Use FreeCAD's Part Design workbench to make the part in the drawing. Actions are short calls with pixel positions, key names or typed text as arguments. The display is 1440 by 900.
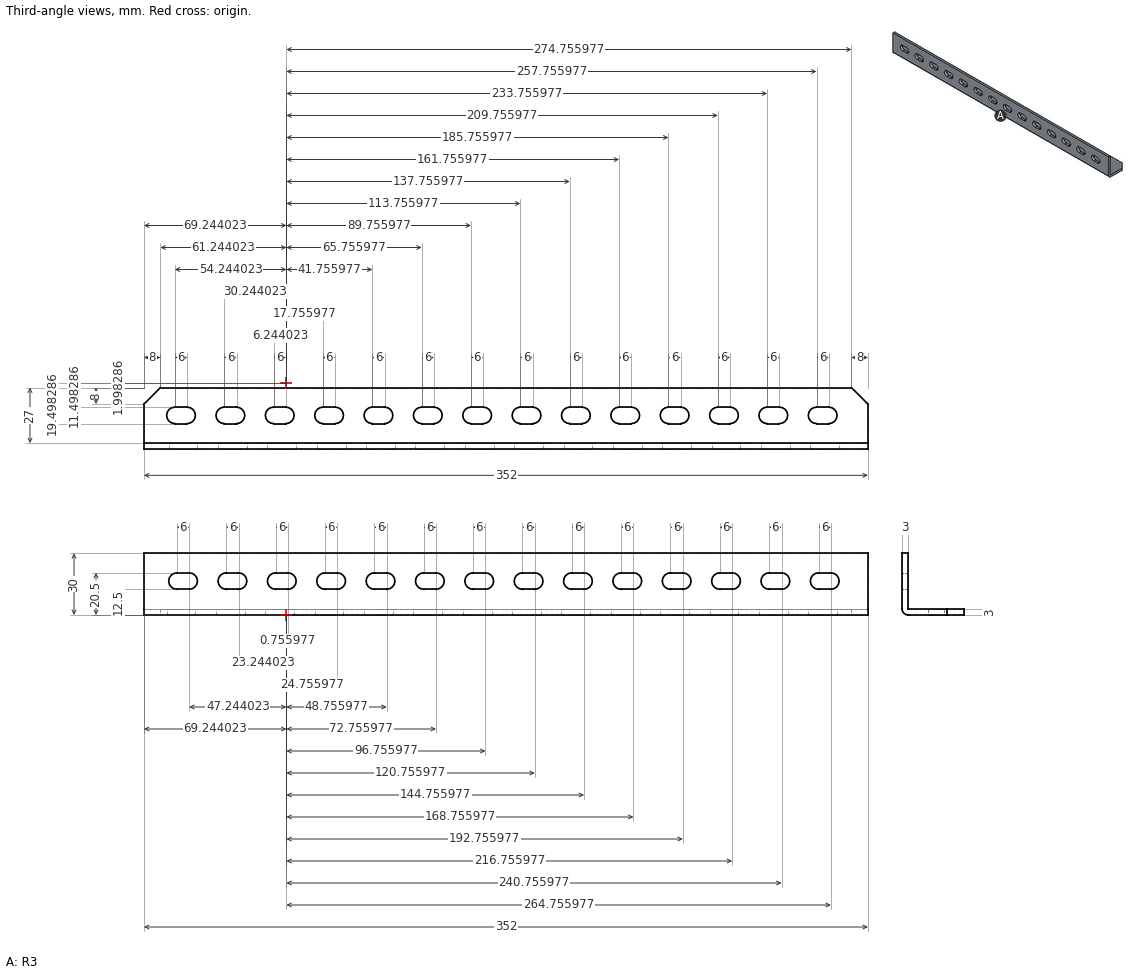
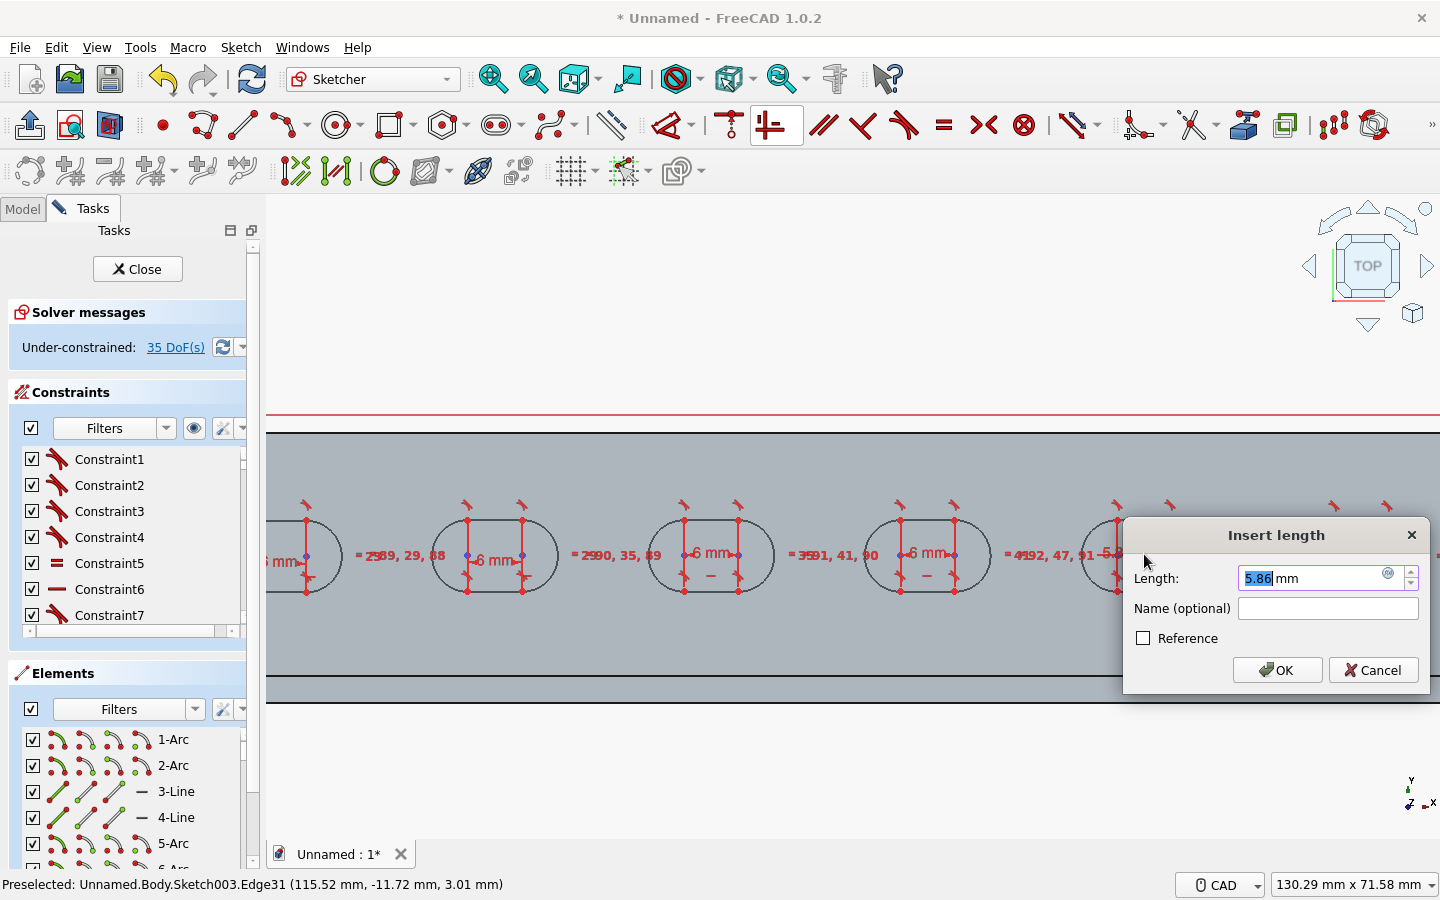
text(6)
key(Return)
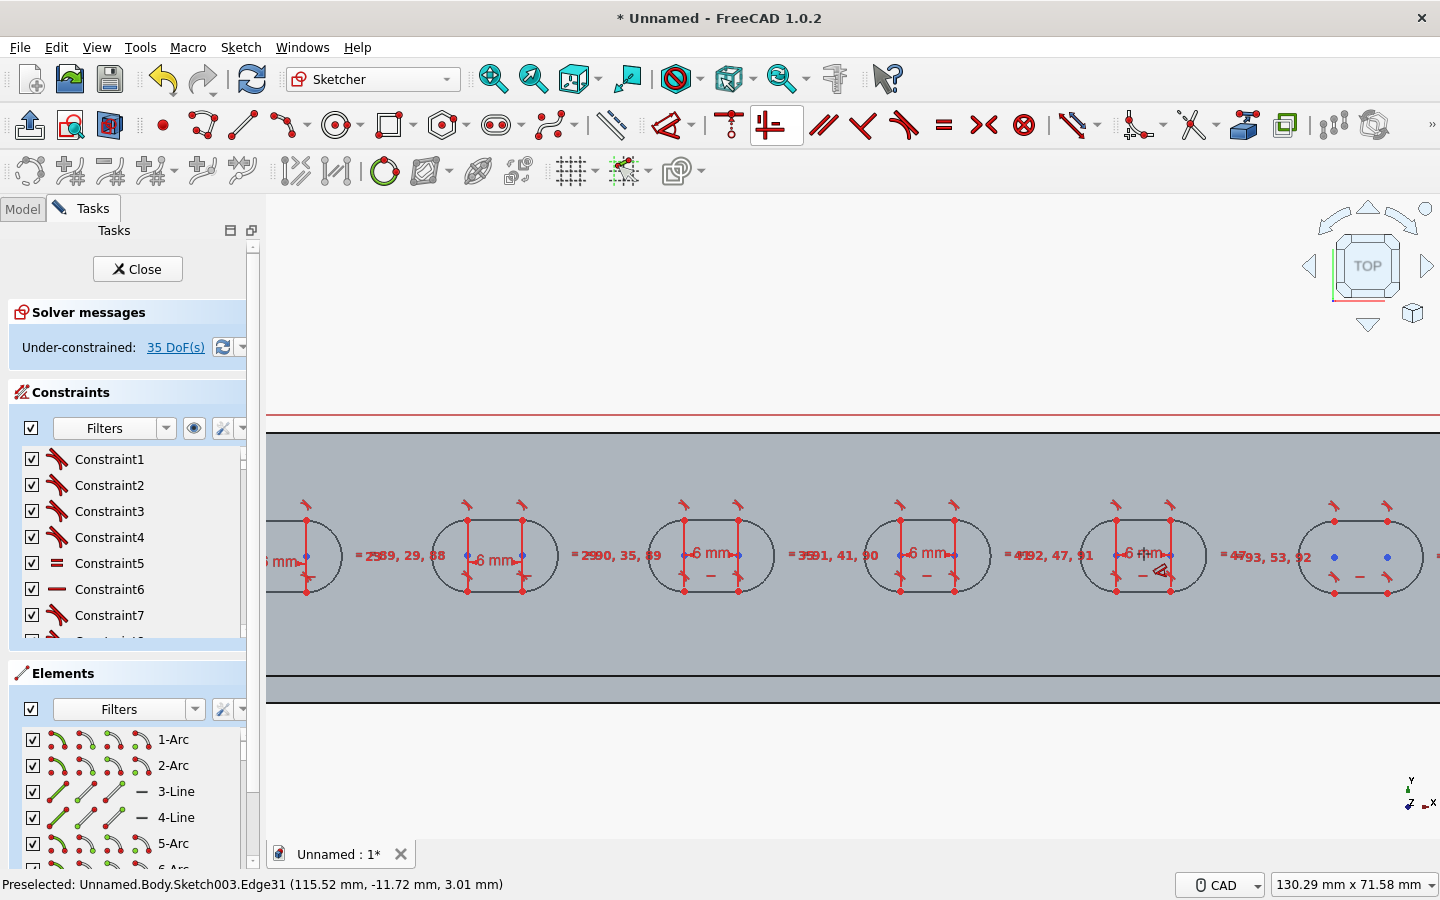
scroll(702, 521, down, 7)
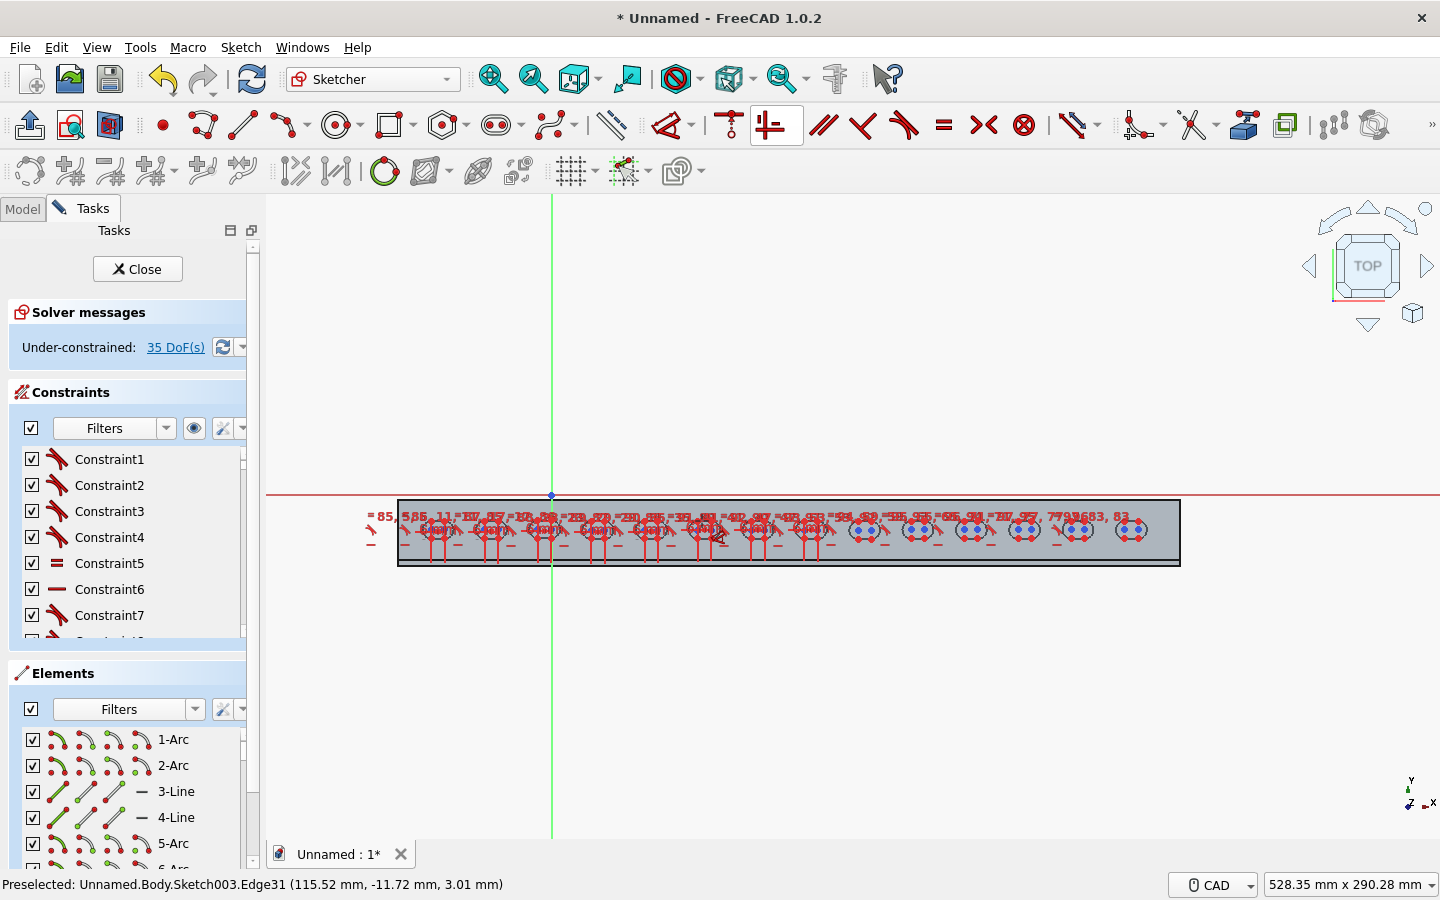
scroll(862, 521, up, 7)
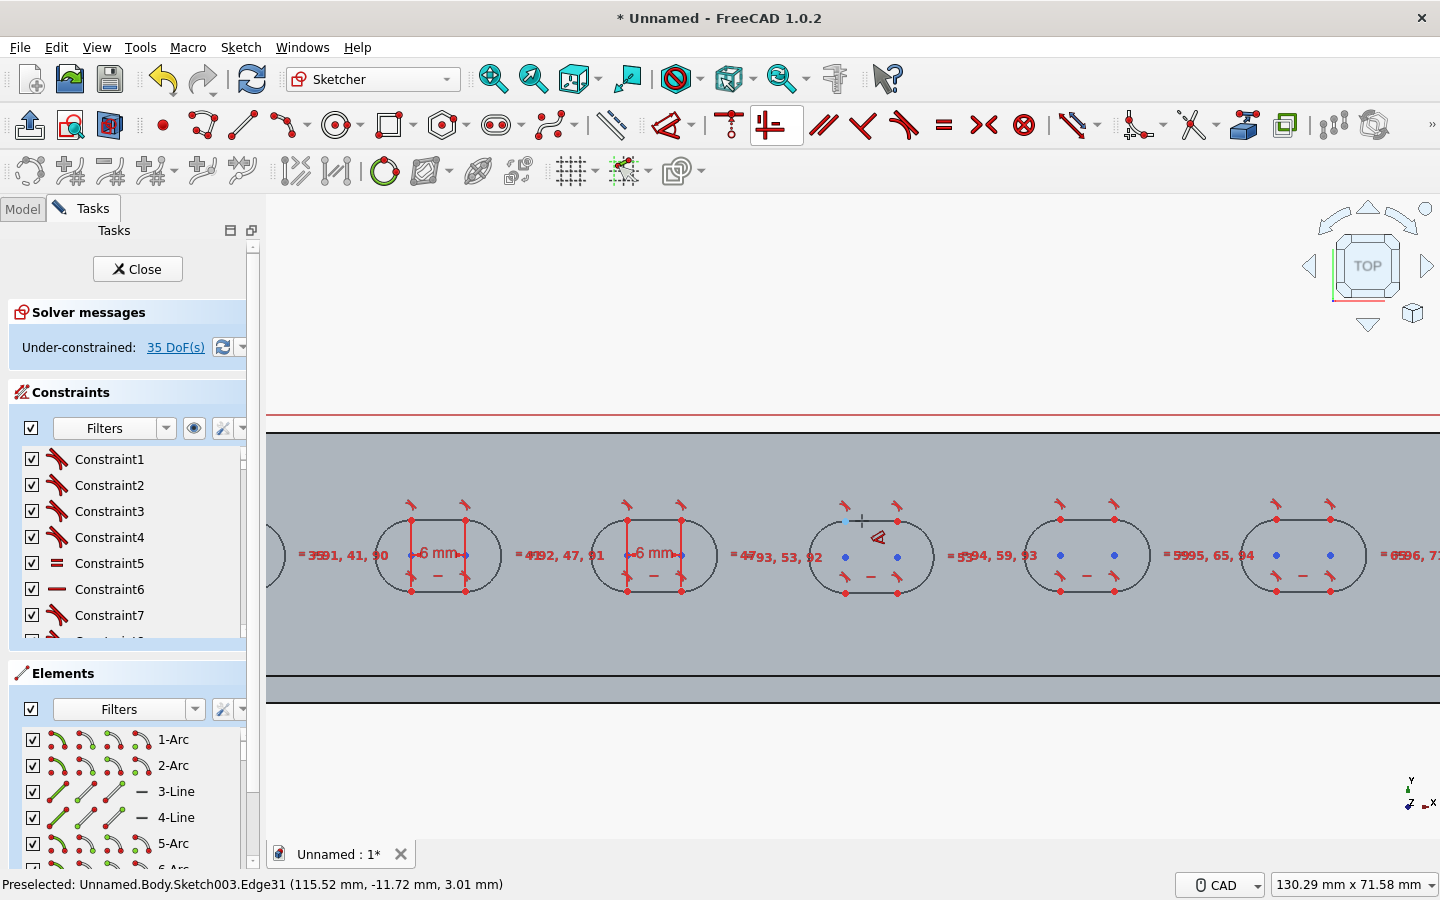
click(861, 521)
click(871, 555)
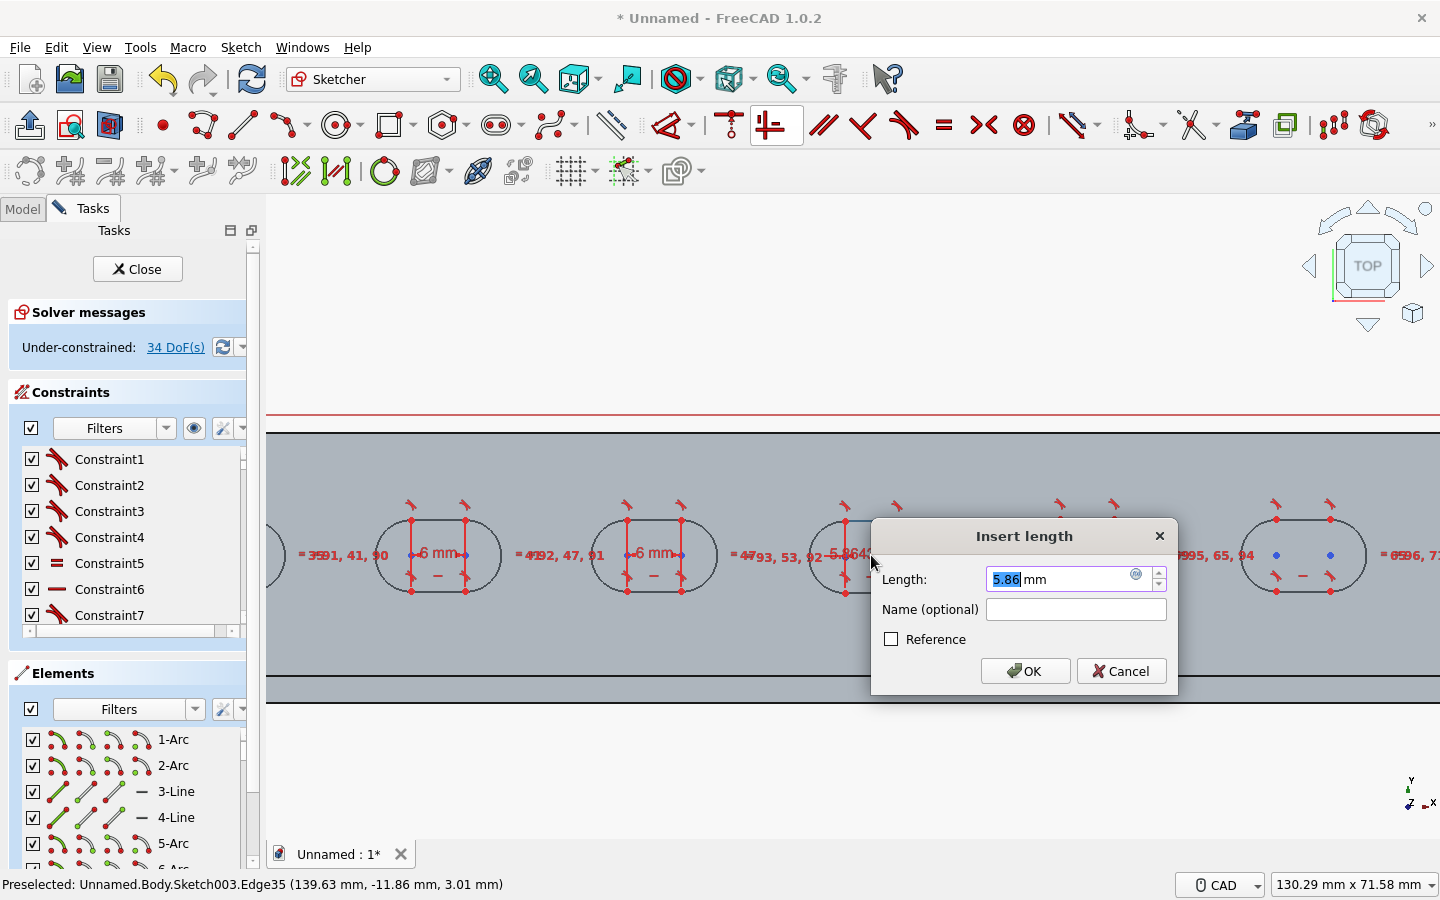
text(6)
key(Return)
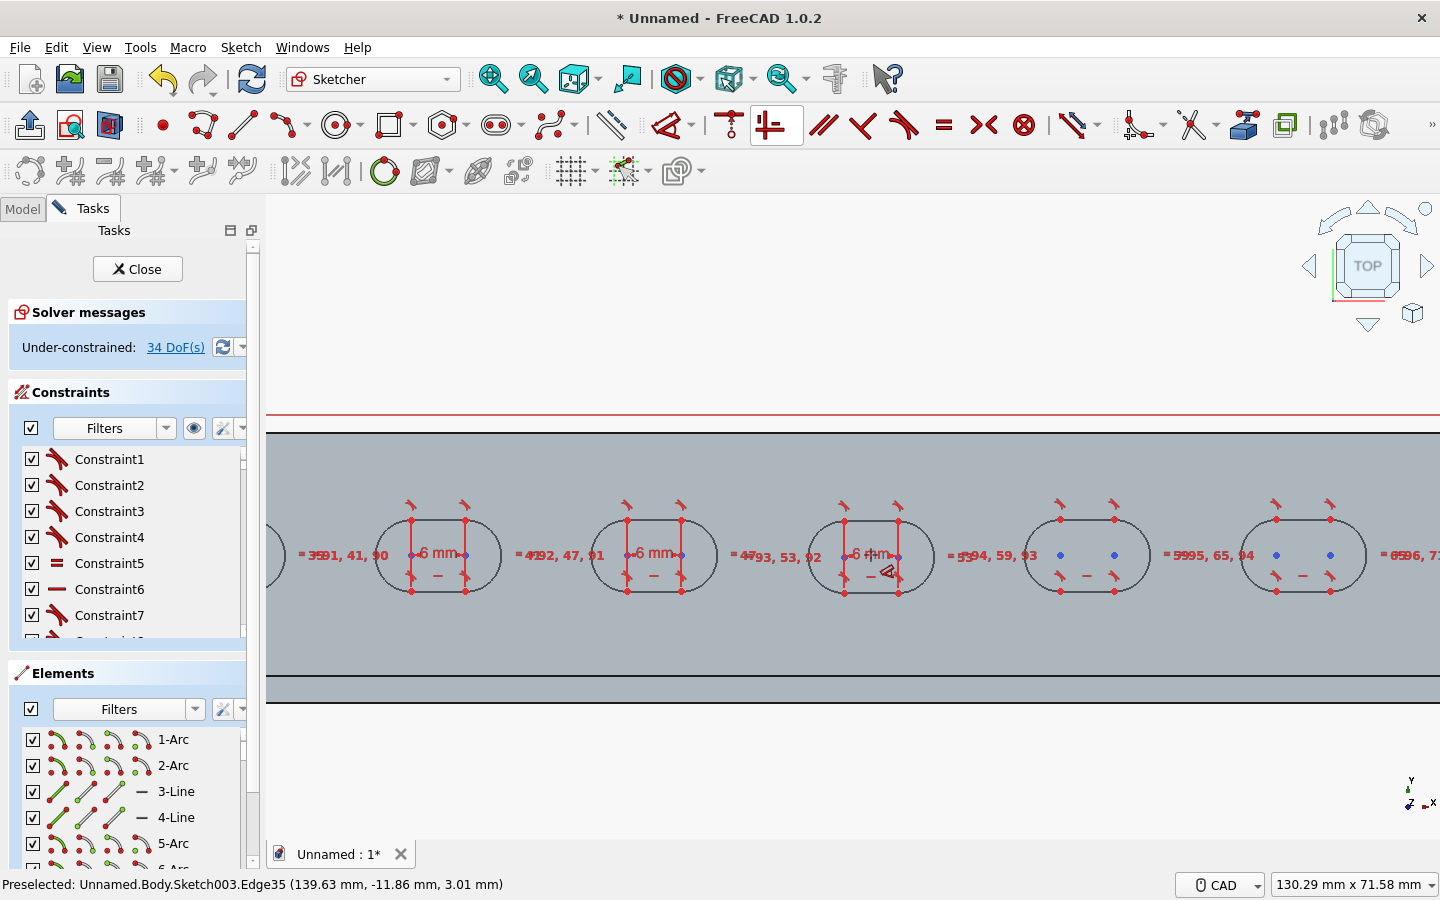
click(1077, 520)
click(1087, 554)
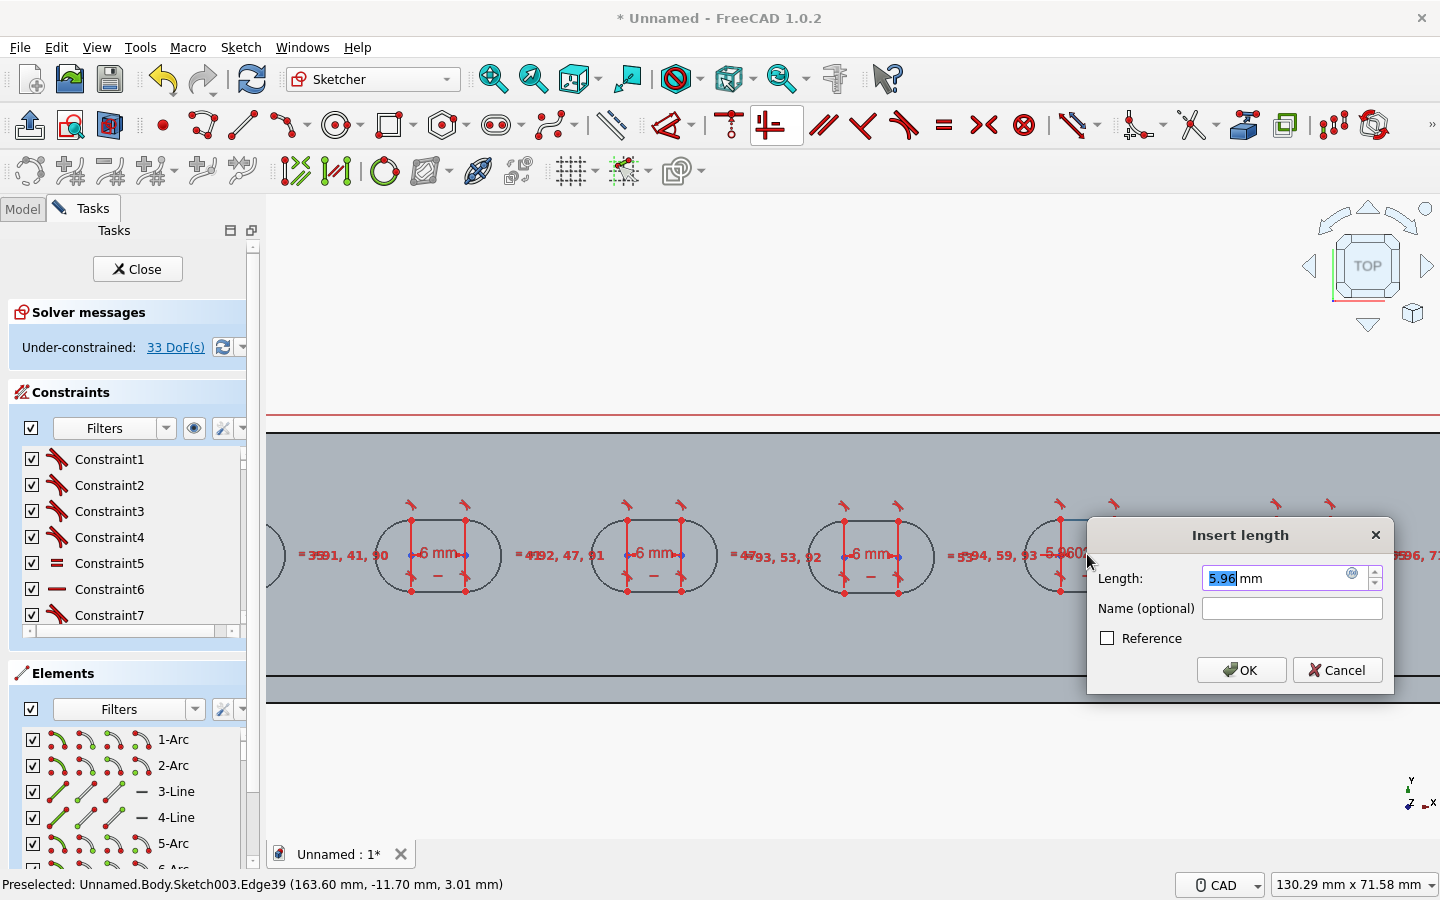
text(6)
key(Return)